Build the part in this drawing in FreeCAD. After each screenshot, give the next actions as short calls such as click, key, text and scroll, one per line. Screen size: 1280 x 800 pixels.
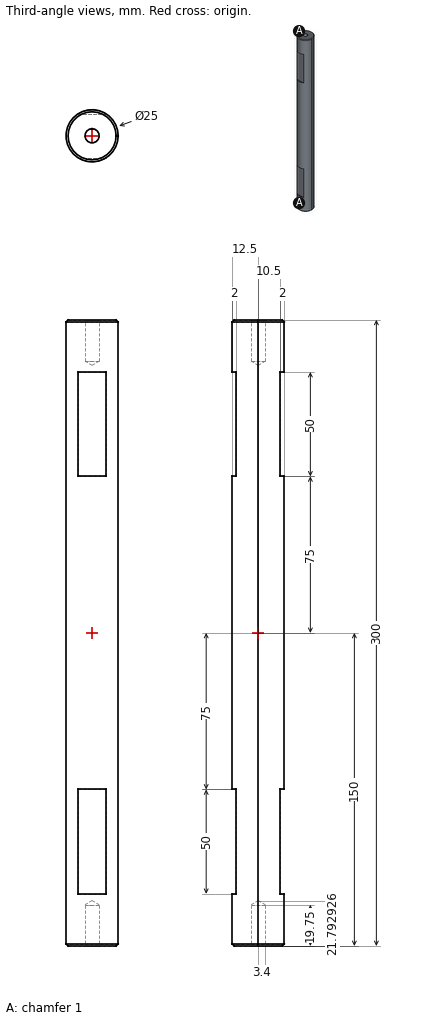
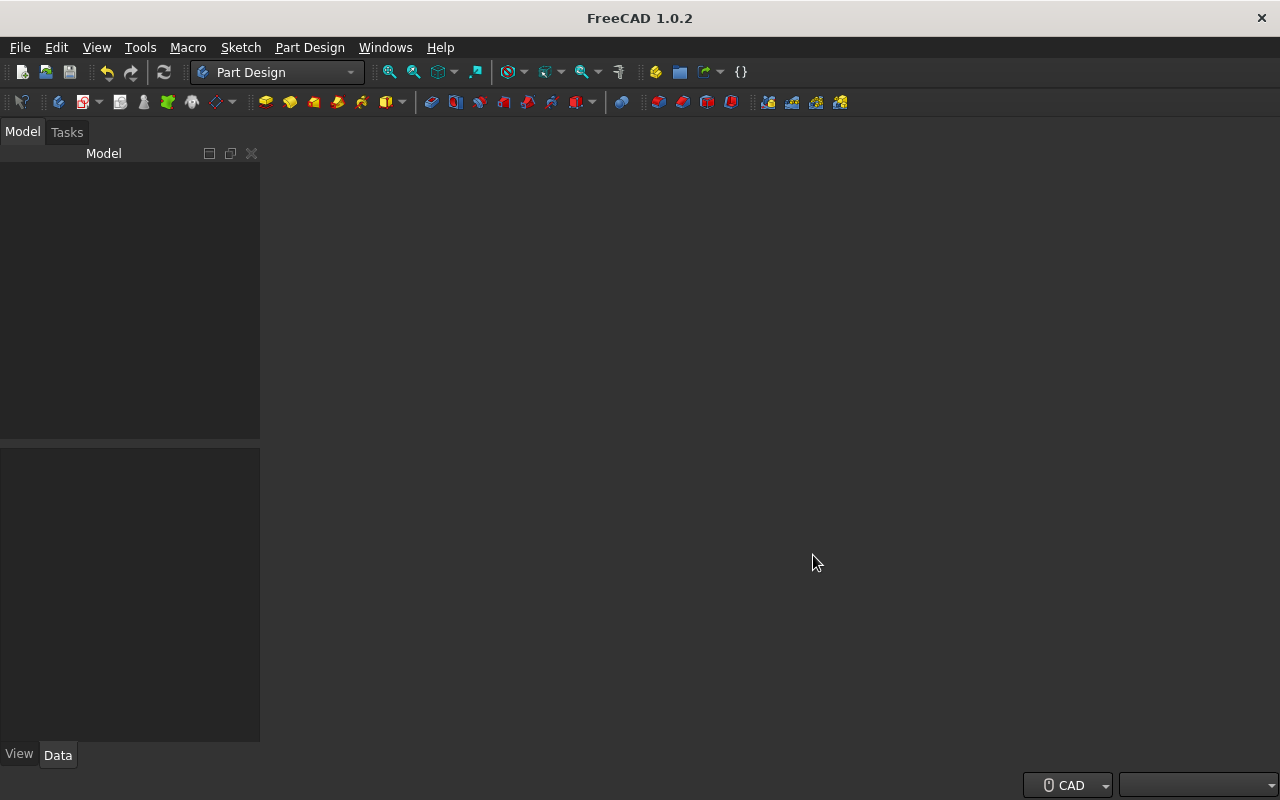
click(22, 72)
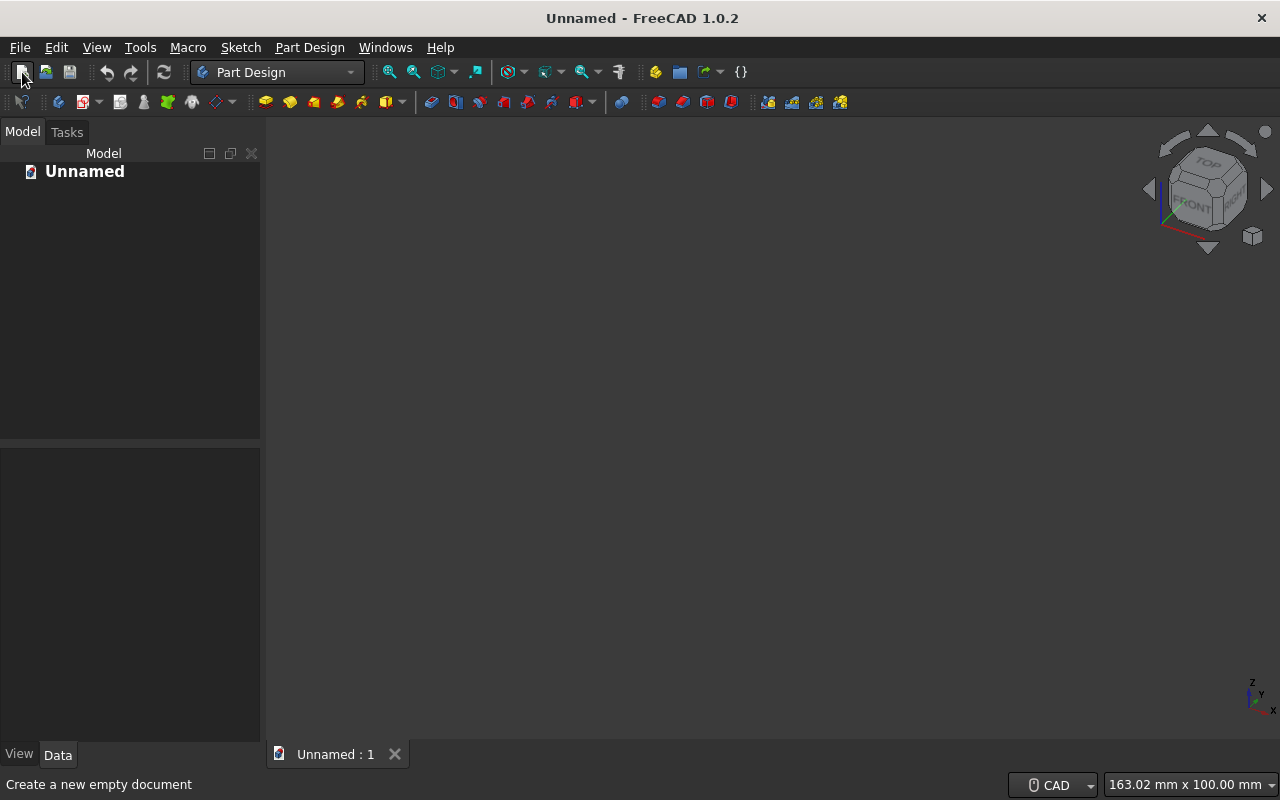
click(84, 102)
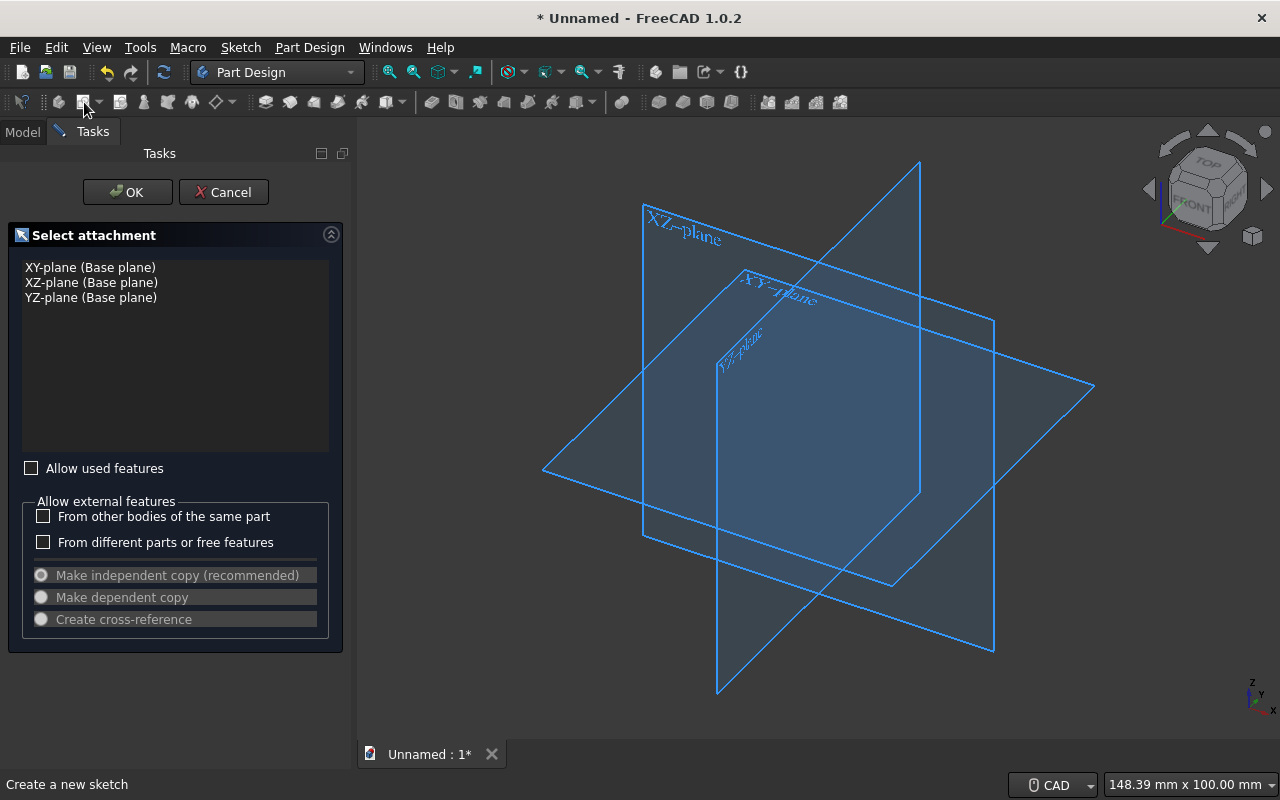
click(82, 268)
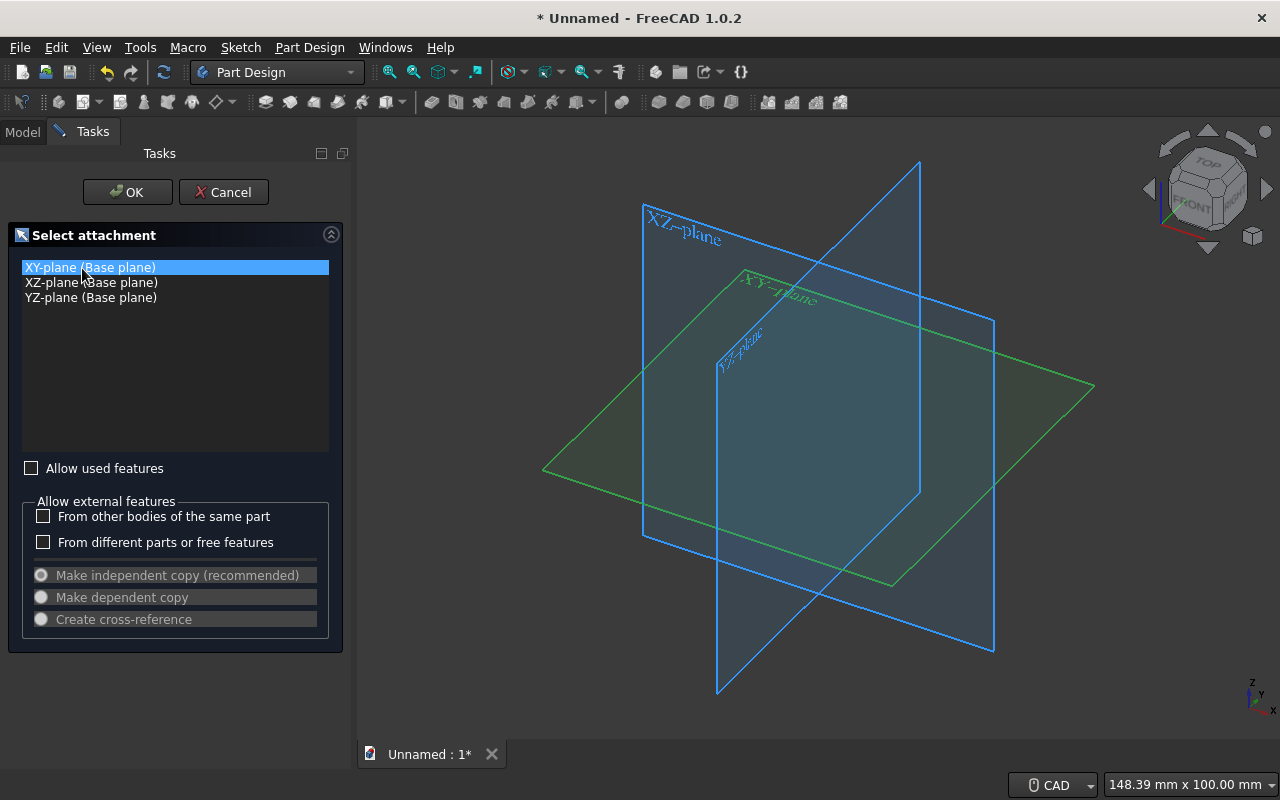
click(128, 192)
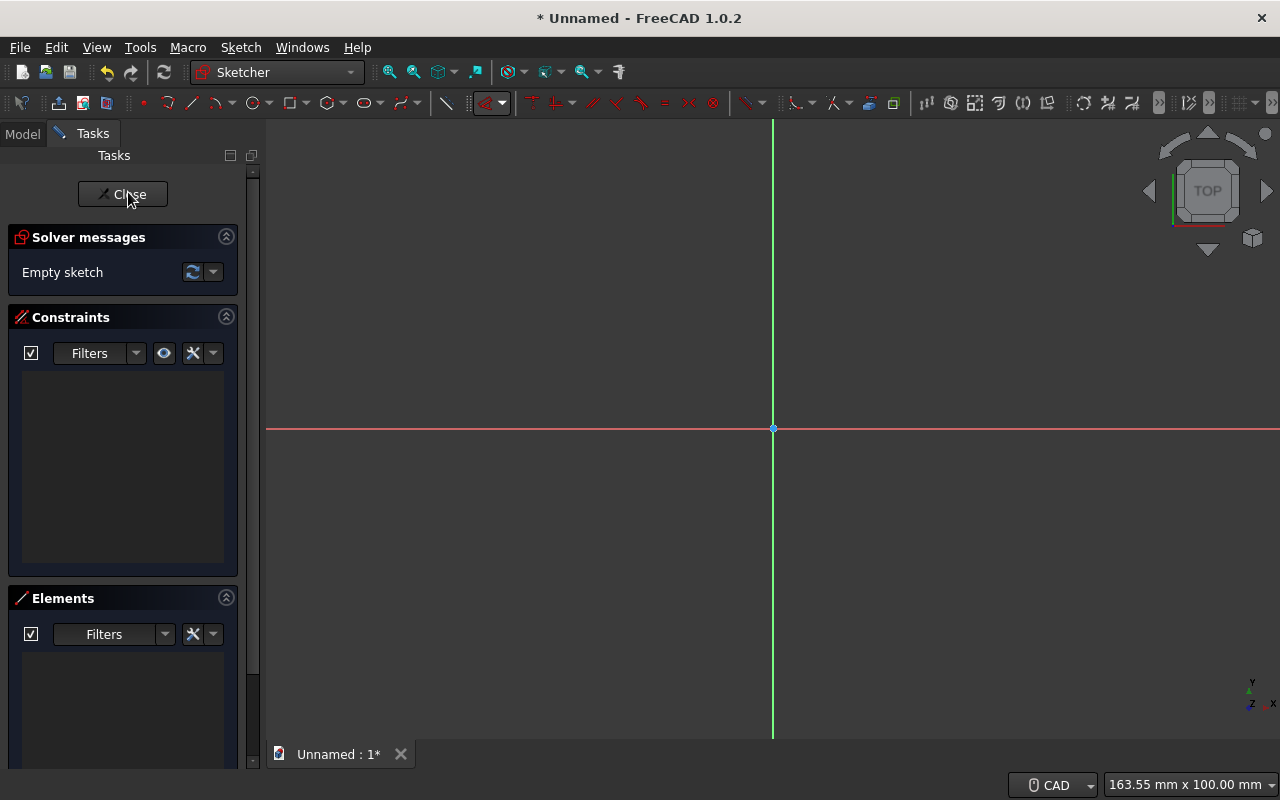
scroll(813, 429, up, 5)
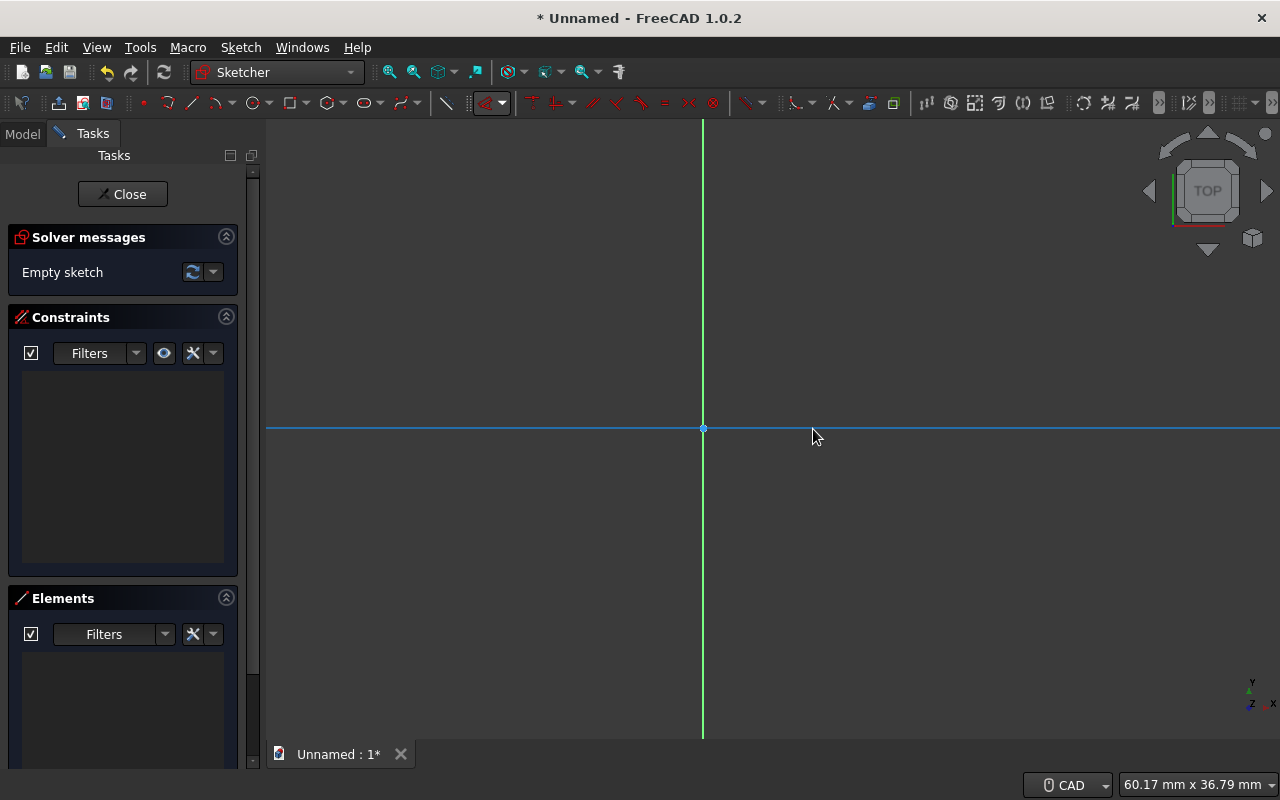
click(254, 104)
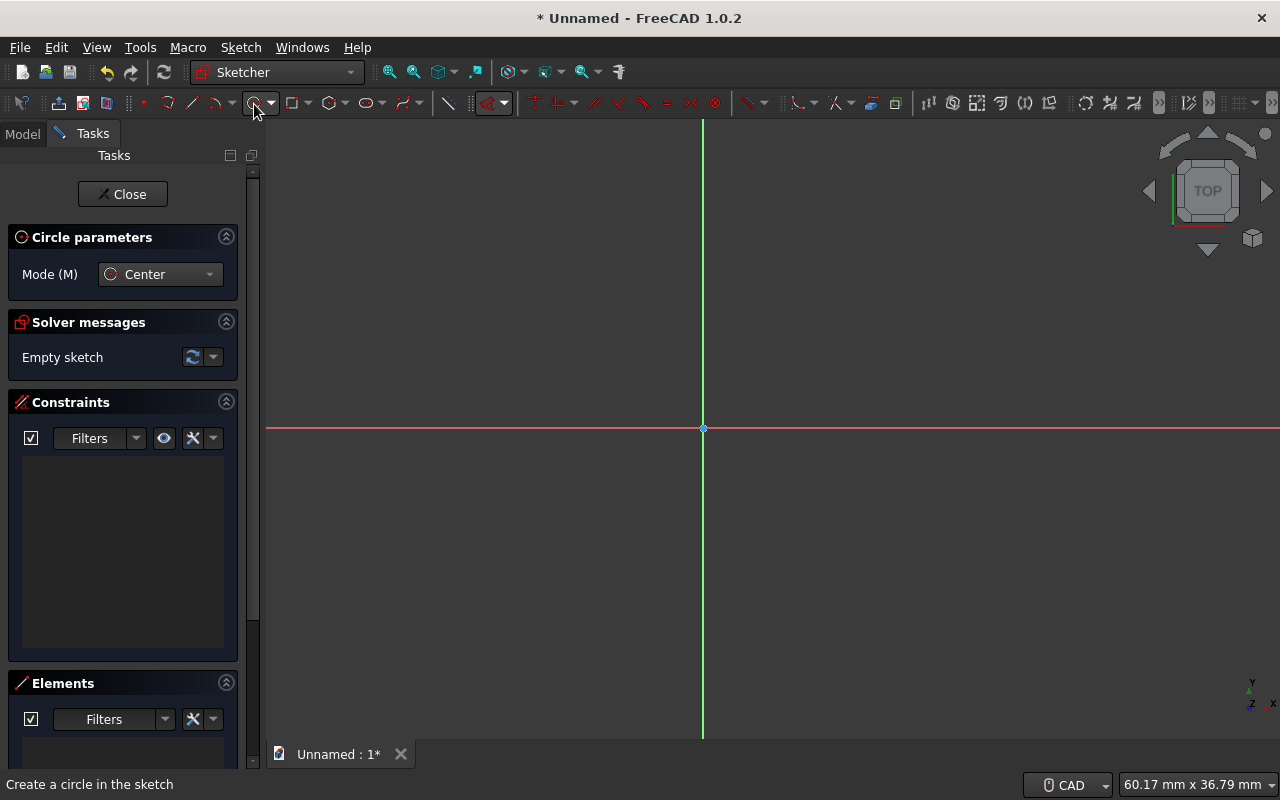
click(703, 428)
move(852, 279)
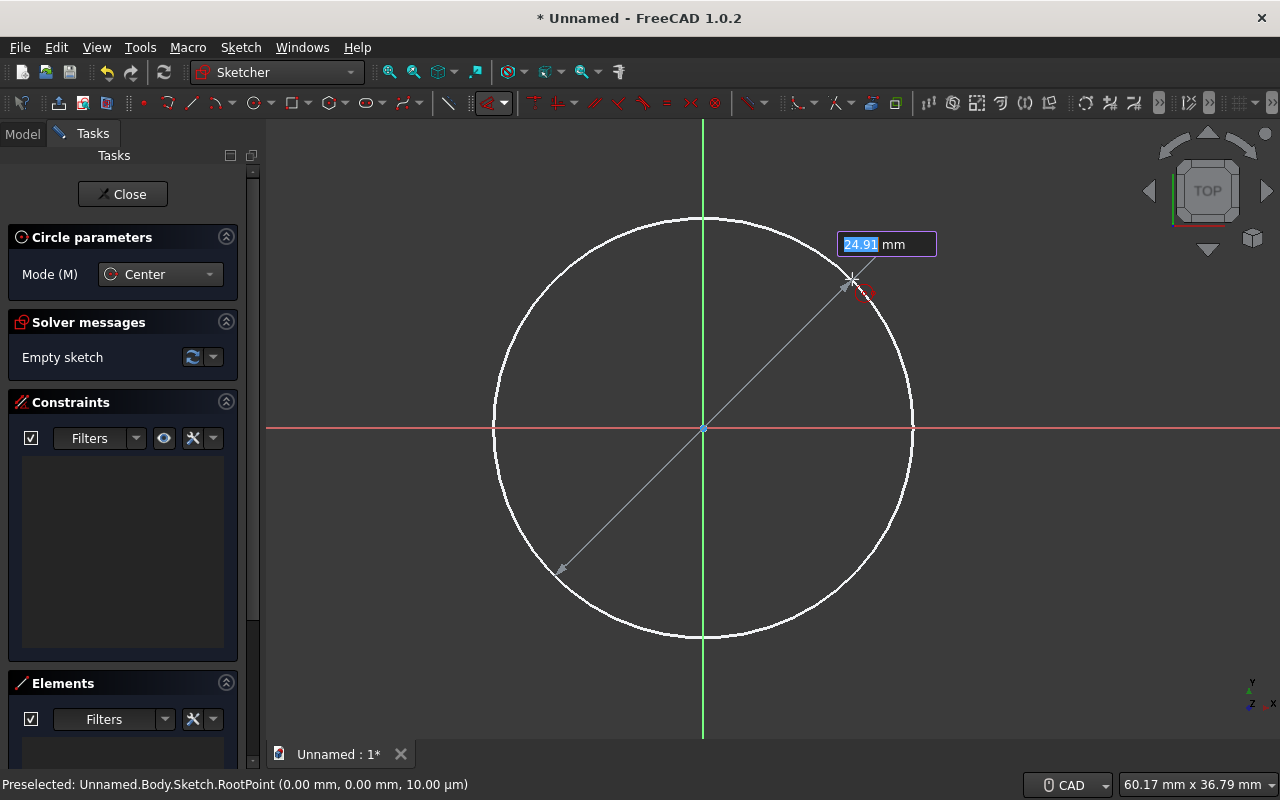
text(25)
key(Return)
key(Escape)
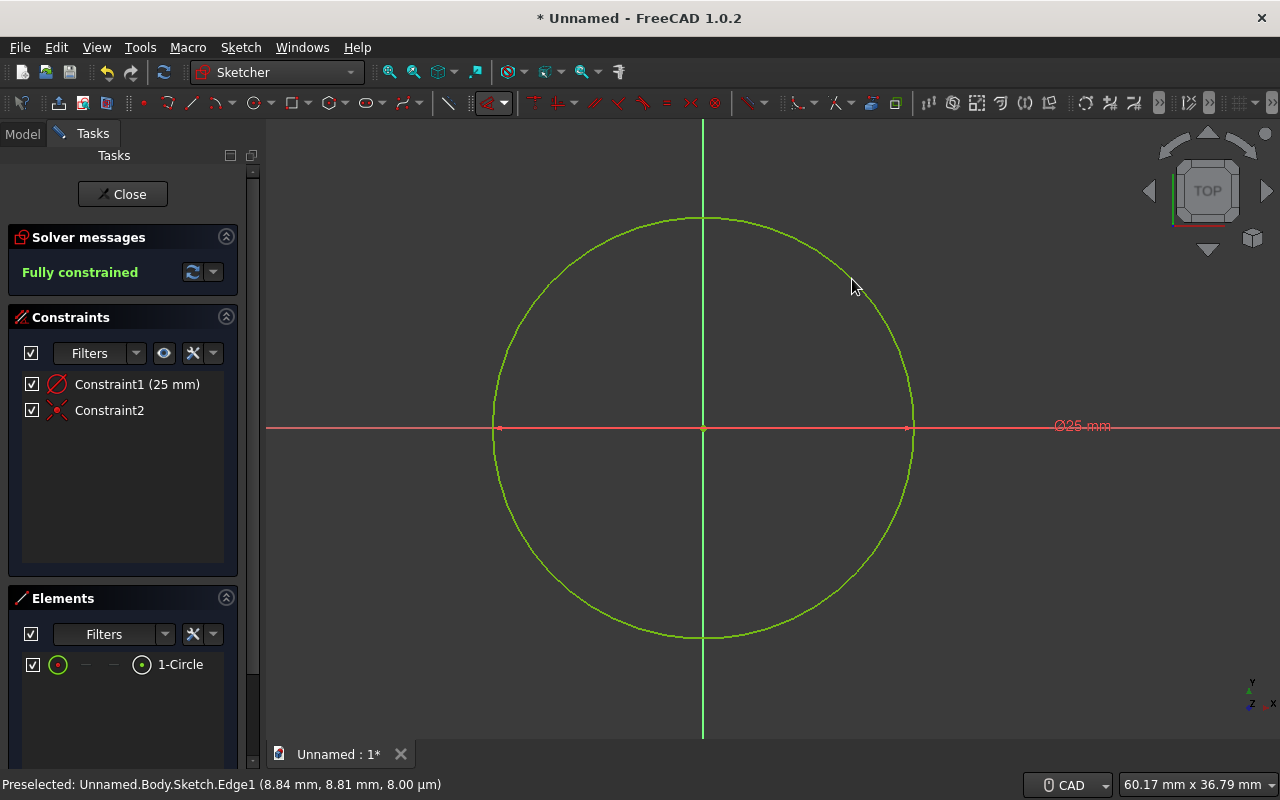
click(123, 194)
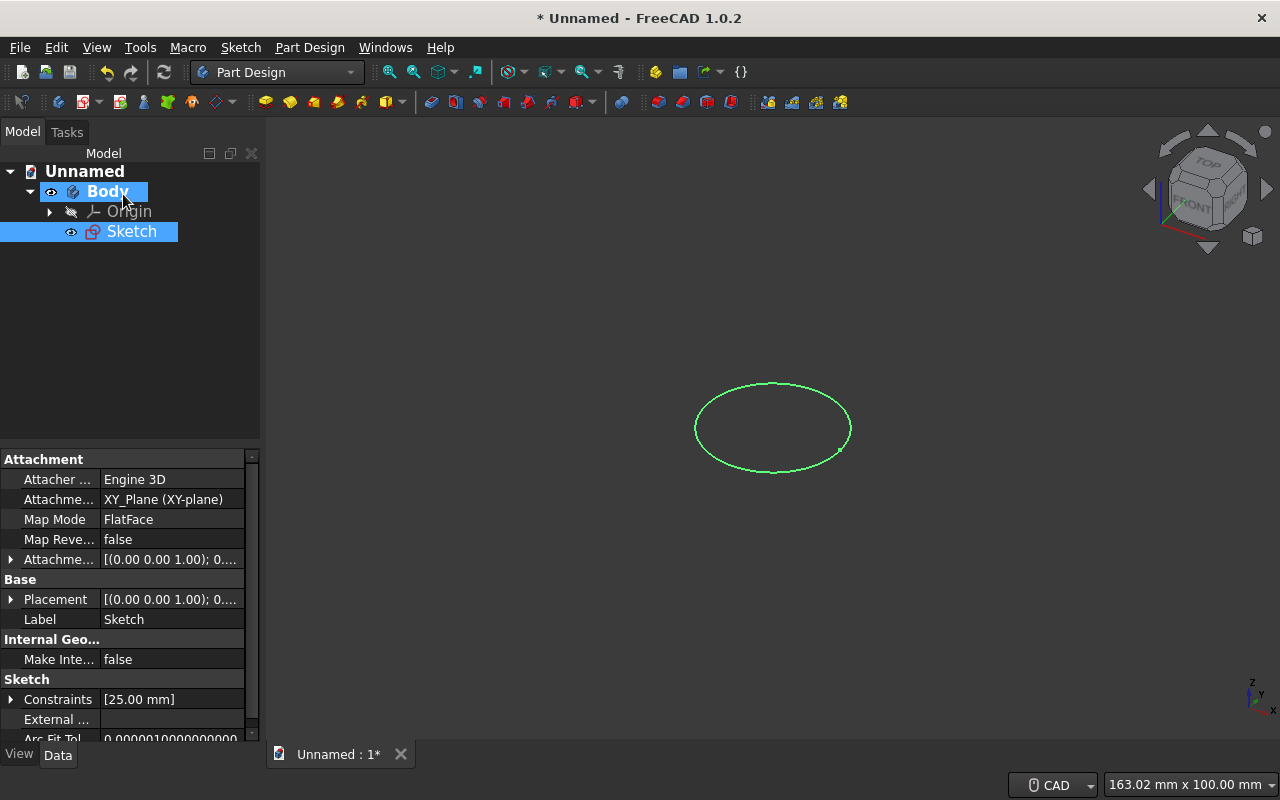
click(266, 102)